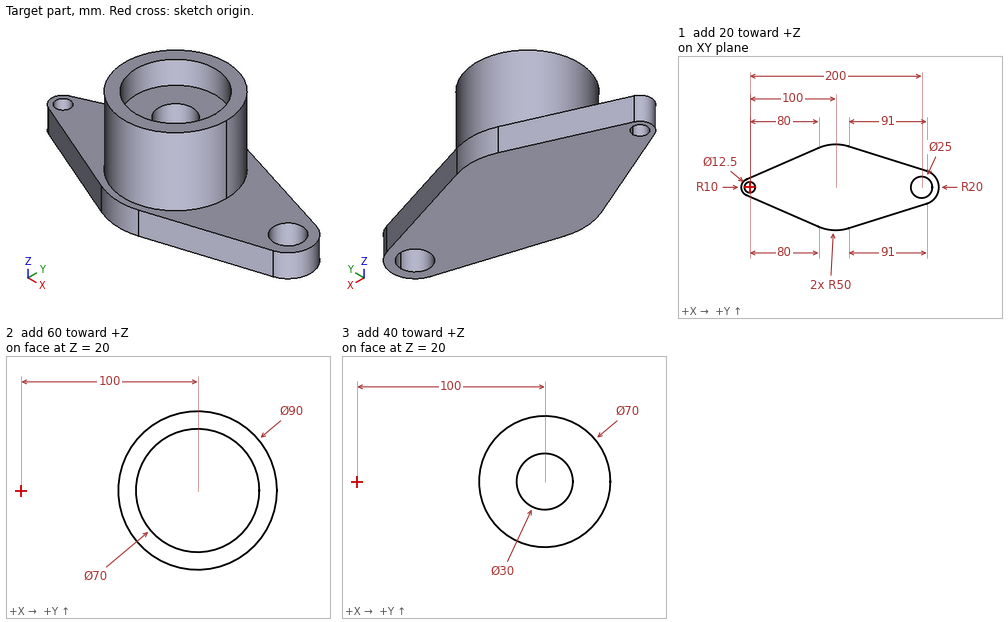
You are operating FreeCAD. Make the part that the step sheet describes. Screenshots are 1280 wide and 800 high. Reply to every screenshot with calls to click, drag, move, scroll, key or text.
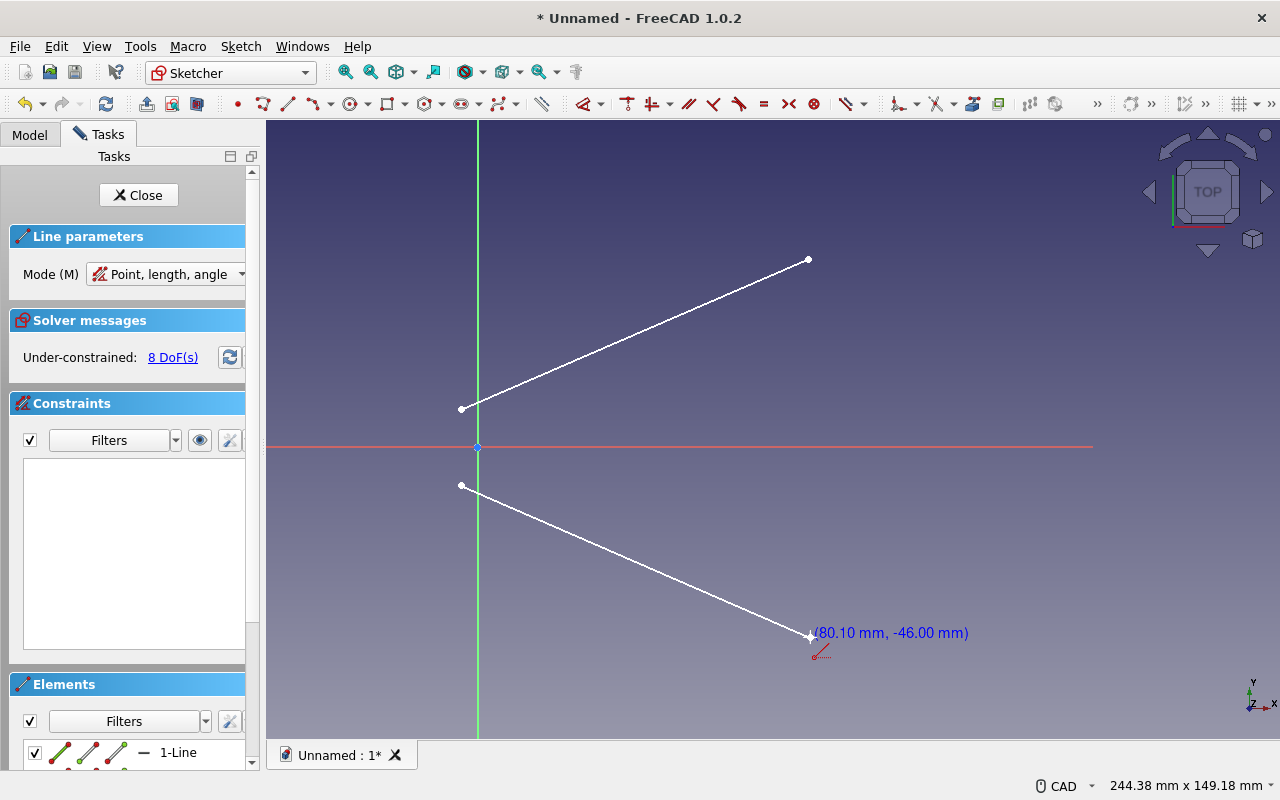
click(955, 645)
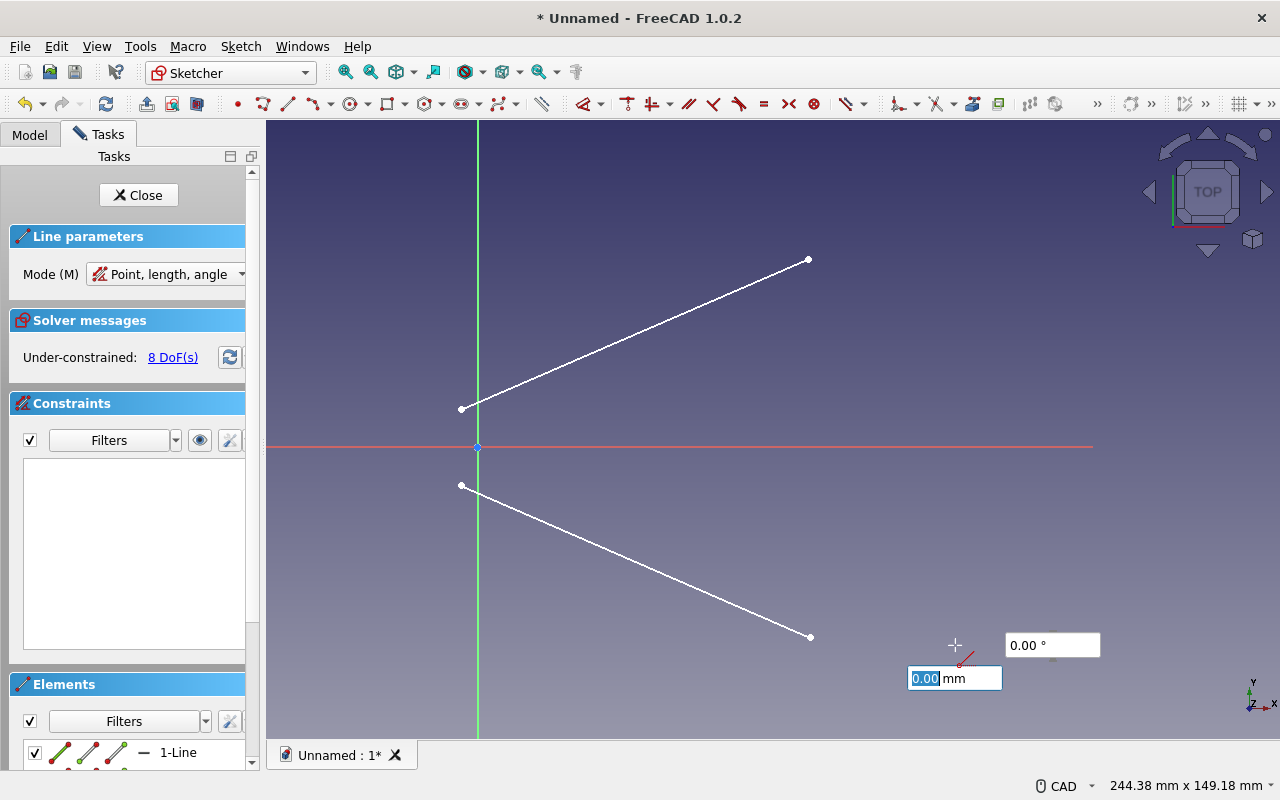
scroll(294, 394, down, 2)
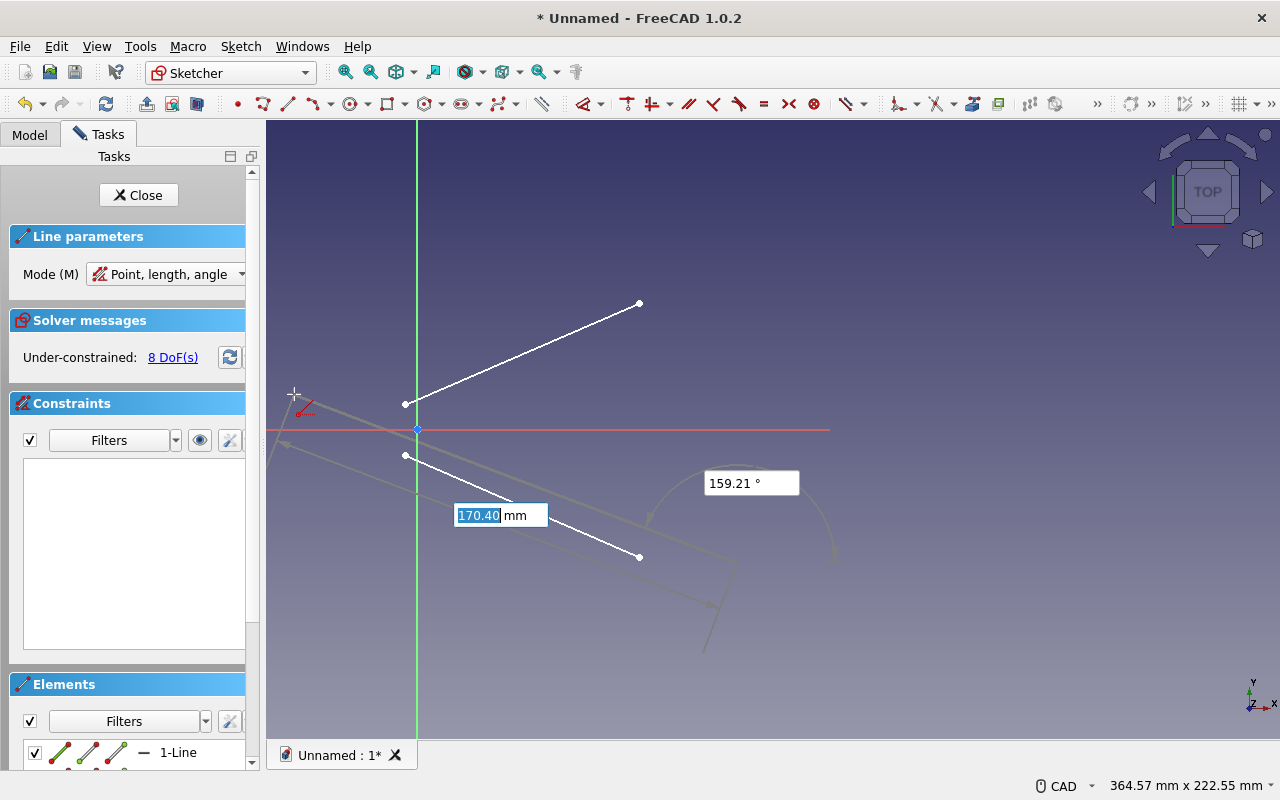
click(990, 483)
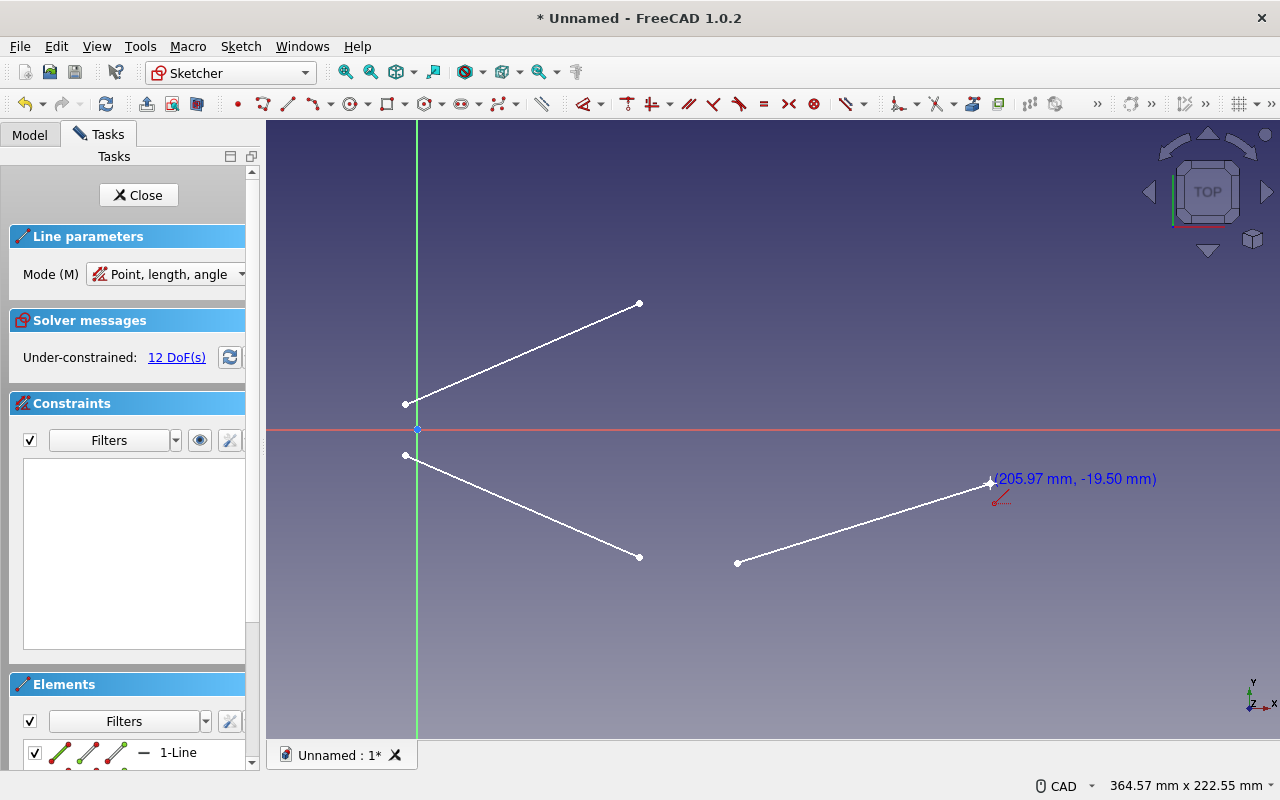
click(990, 377)
click(737, 297)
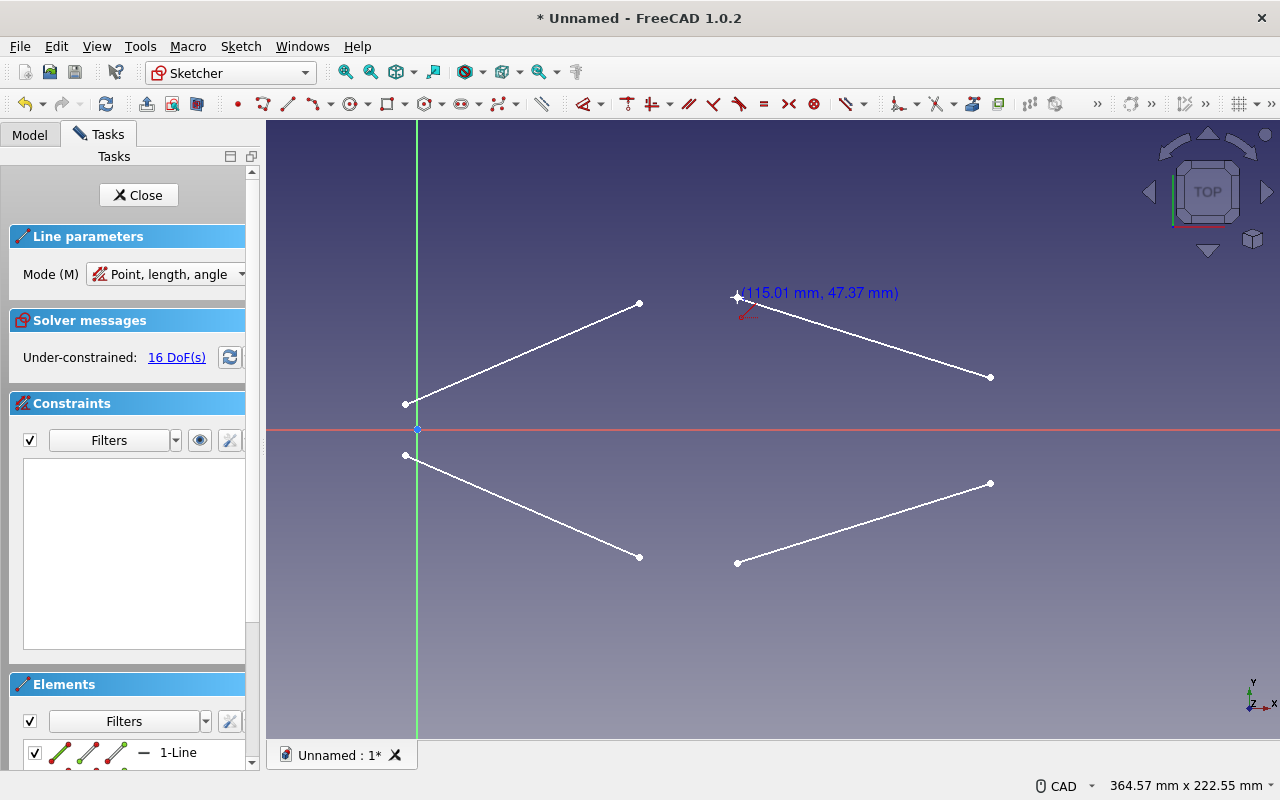
click(312, 104)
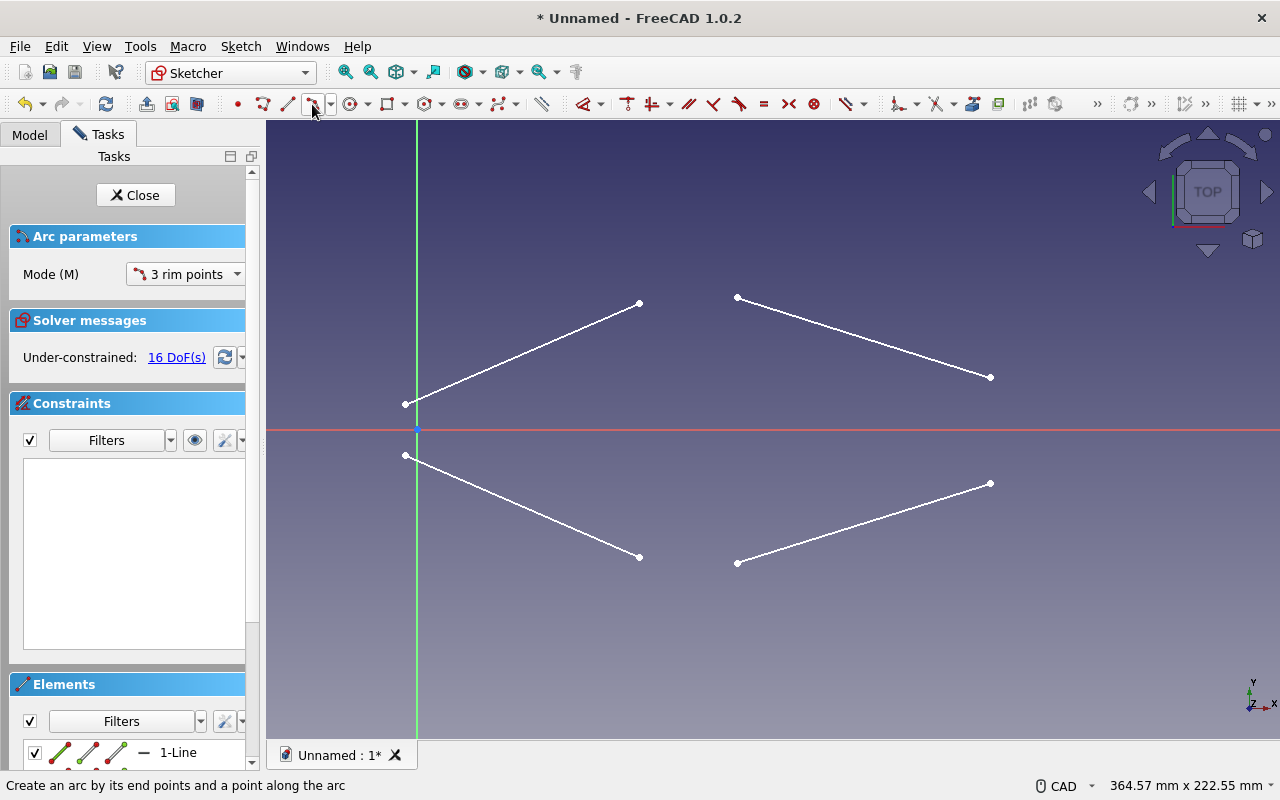
scroll(406, 404, up, 2)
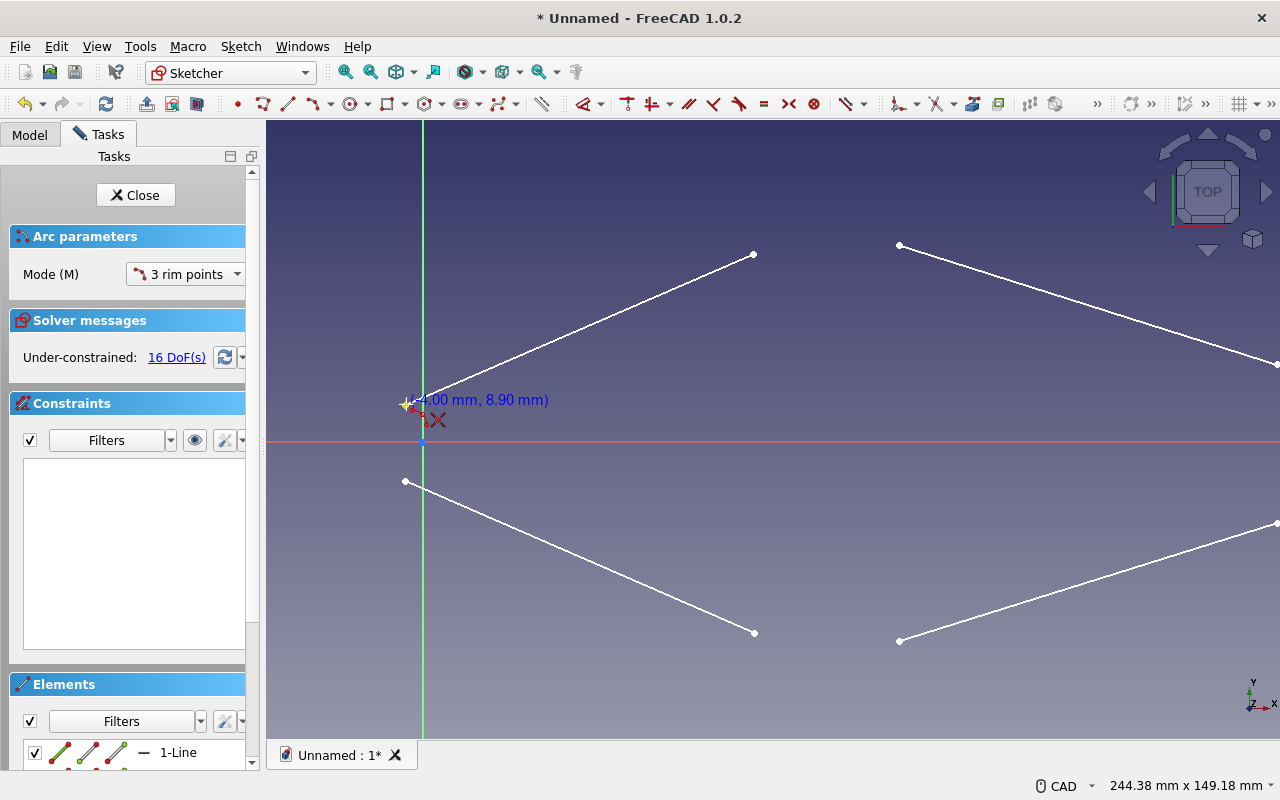
click(406, 405)
click(406, 481)
click(385, 424)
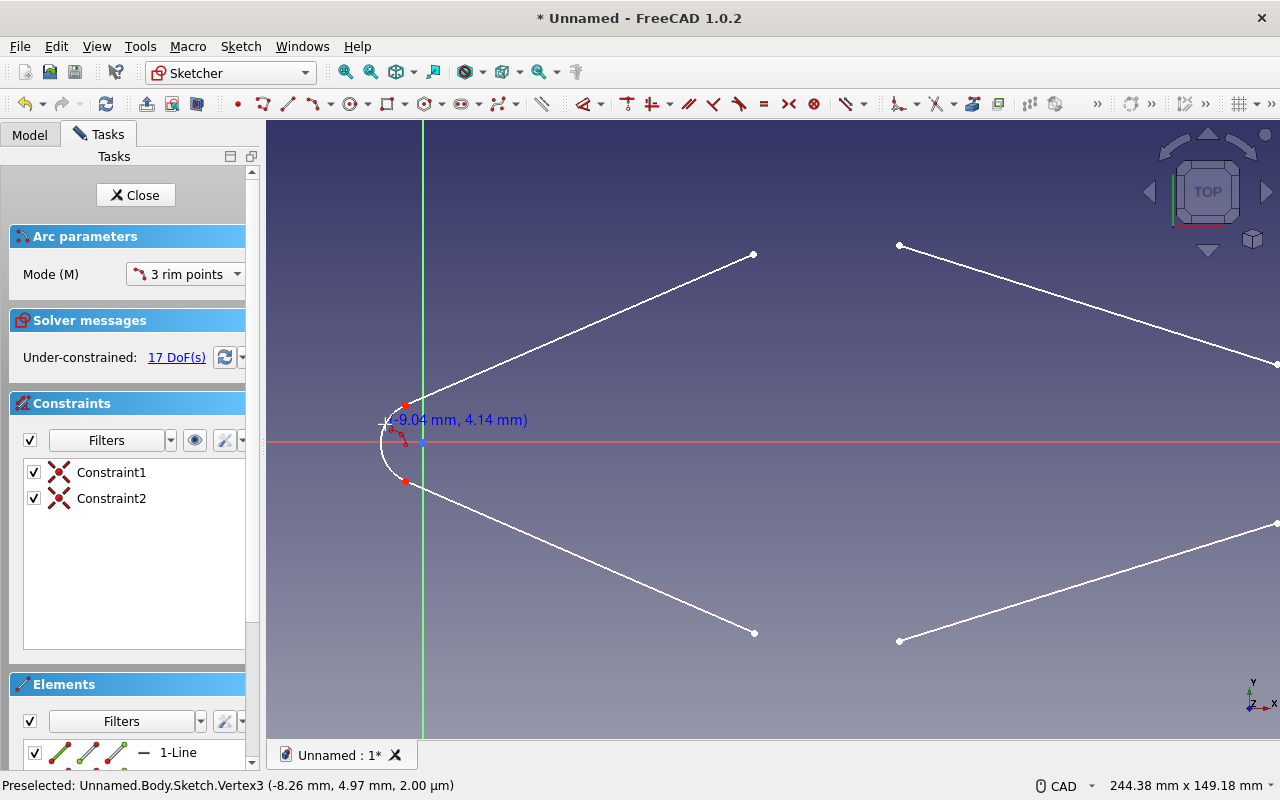
click(755, 633)
click(900, 641)
click(826, 649)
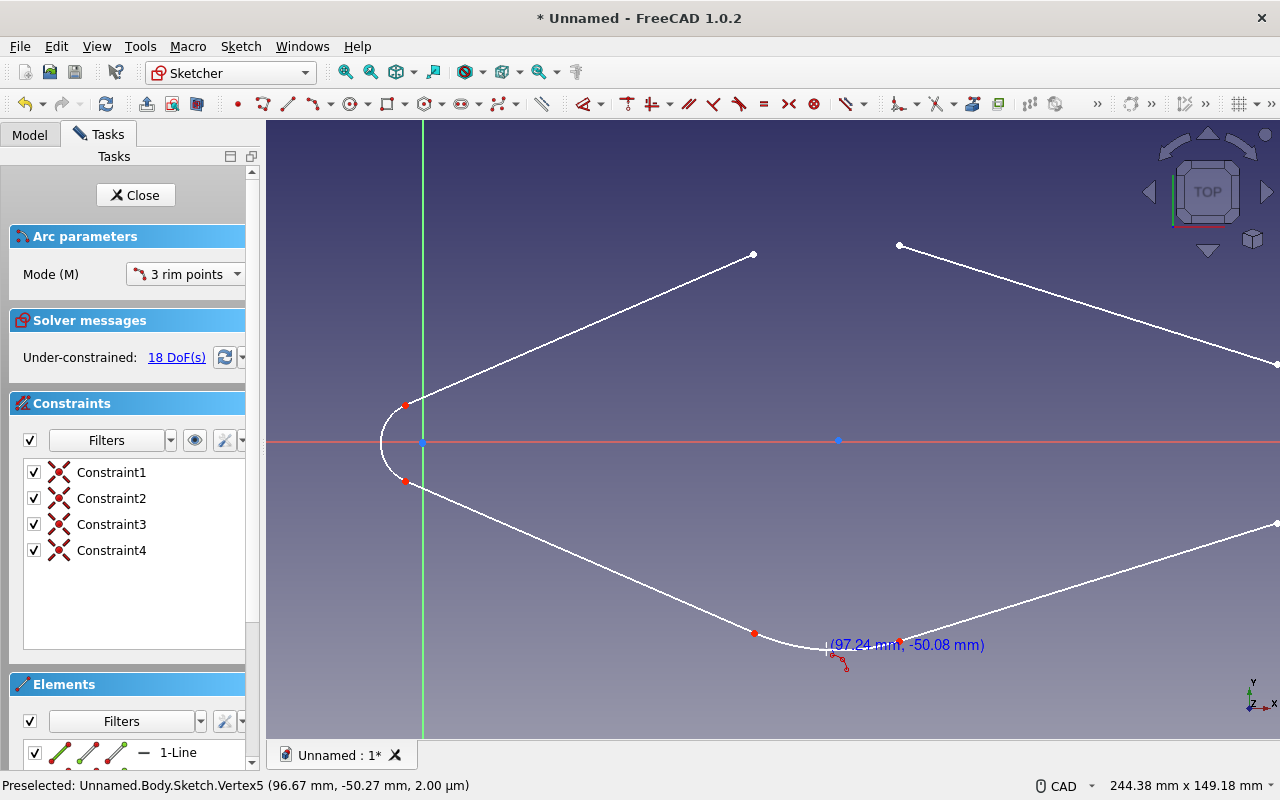
scroll(392, 404, down, 2)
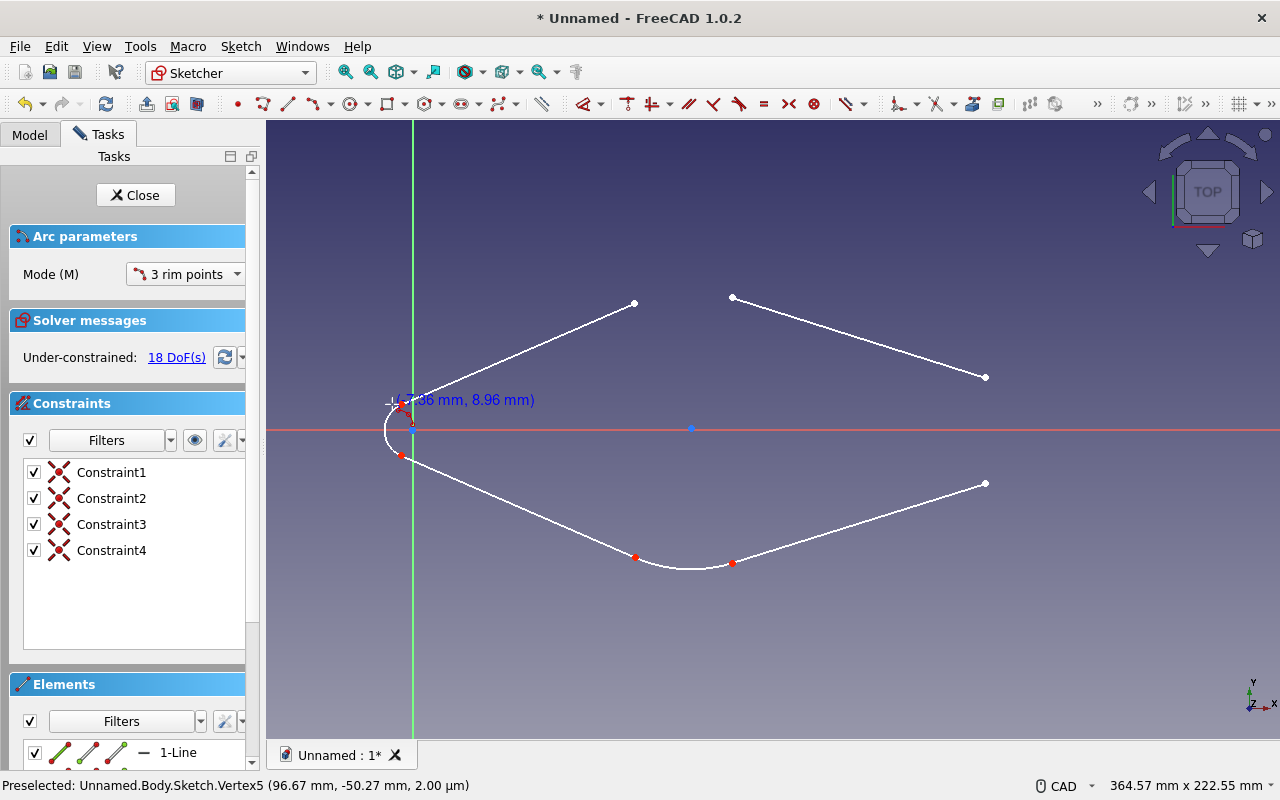
click(985, 484)
click(985, 378)
click(1017, 457)